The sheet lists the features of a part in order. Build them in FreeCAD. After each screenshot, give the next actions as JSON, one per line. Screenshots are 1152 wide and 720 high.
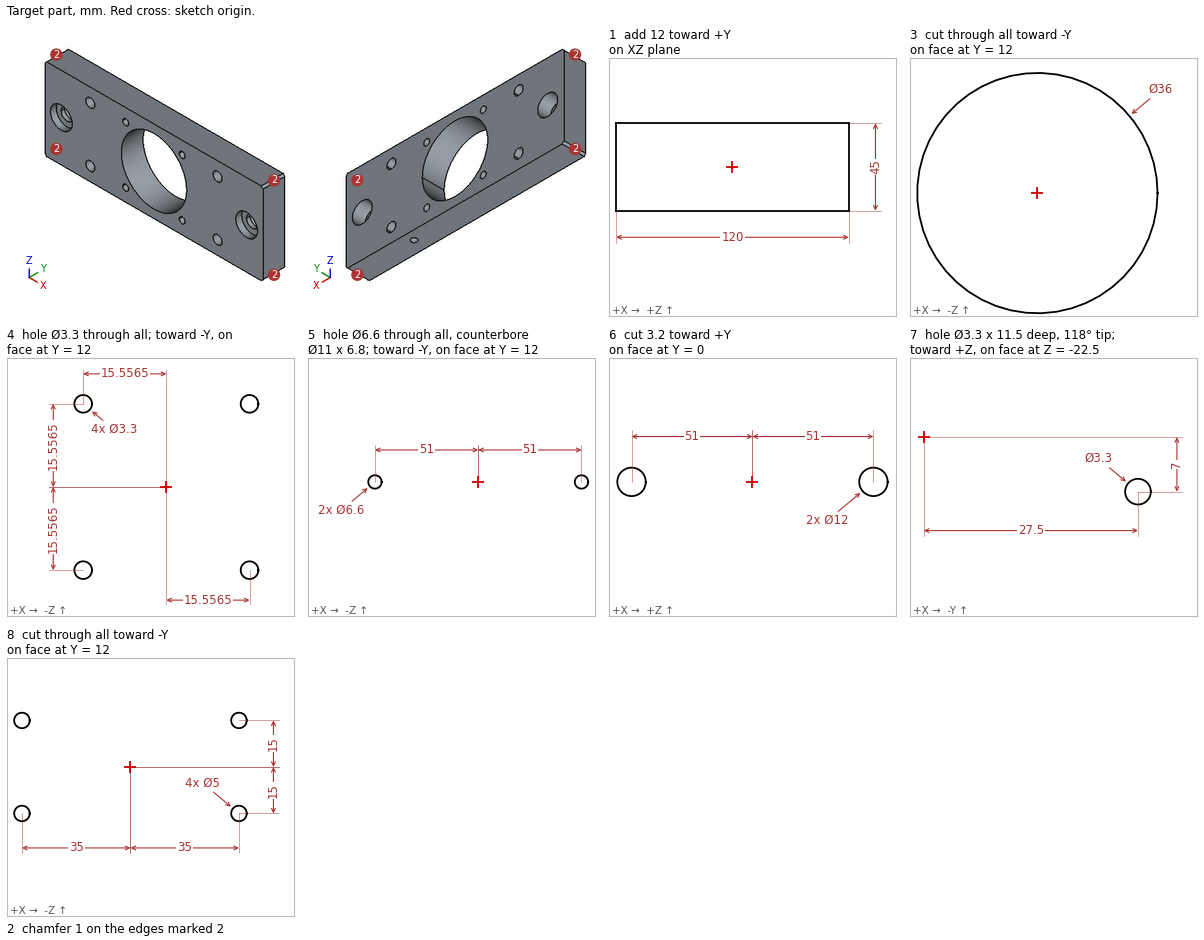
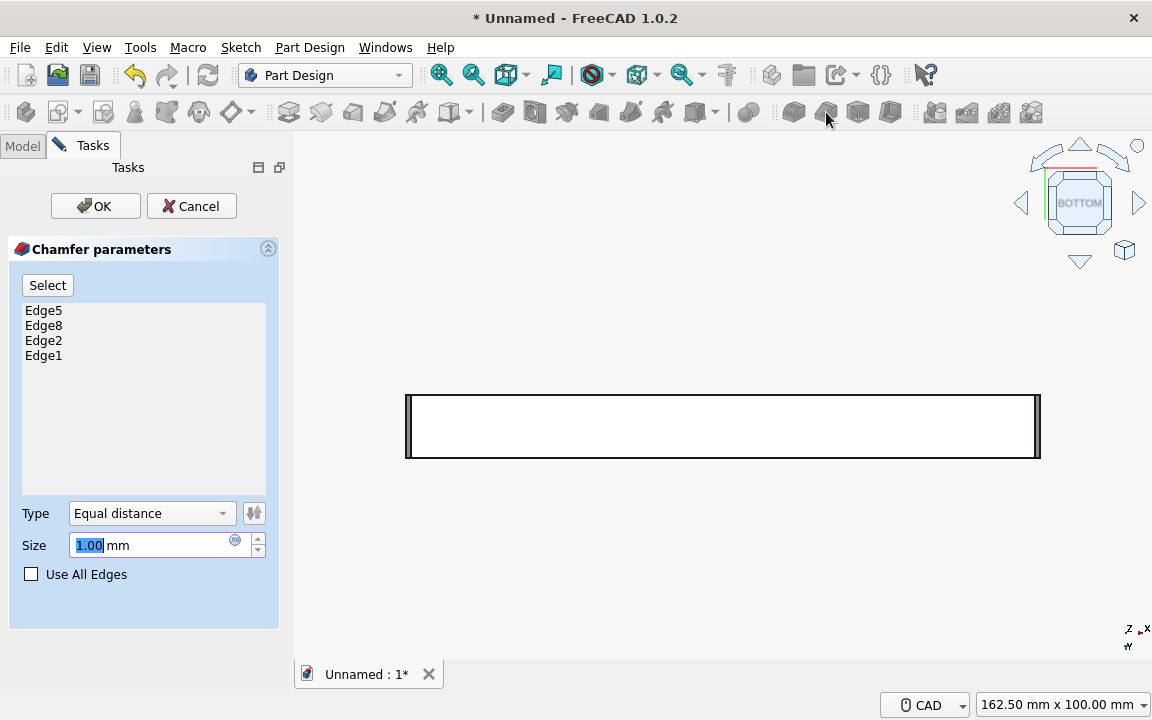
{"action": "type", "text": "1"}
{"action": "key", "text": "Tab"}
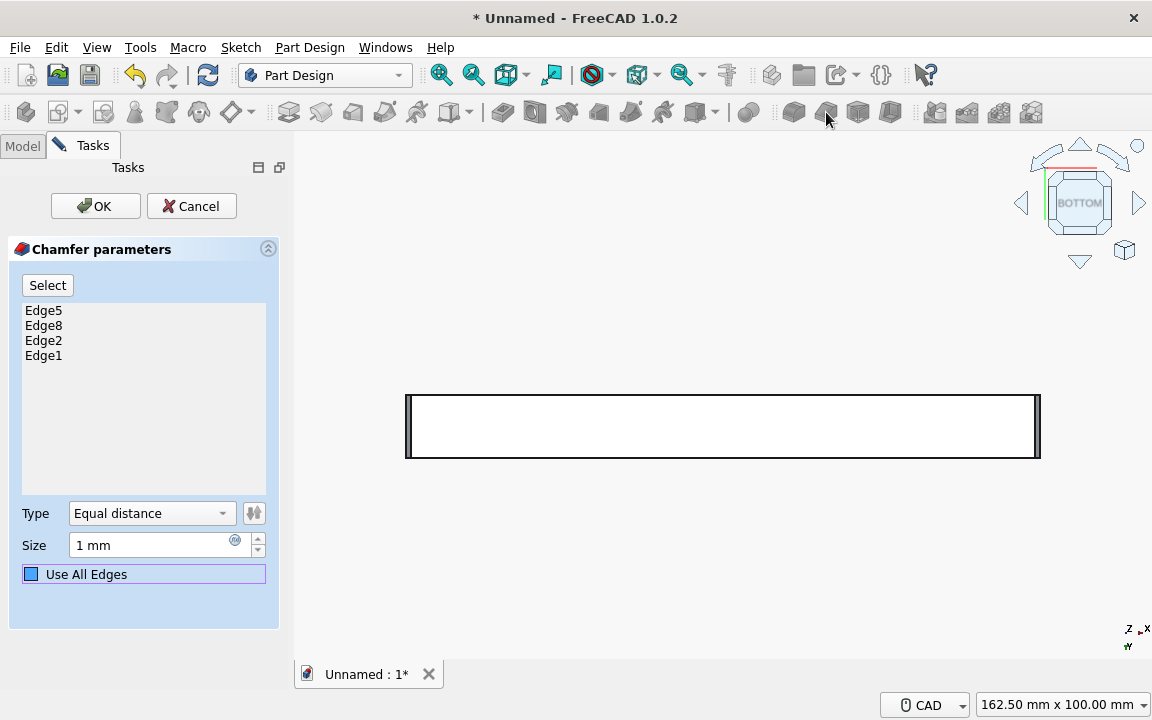
{"action": "left_click", "coordinate": [96, 206]}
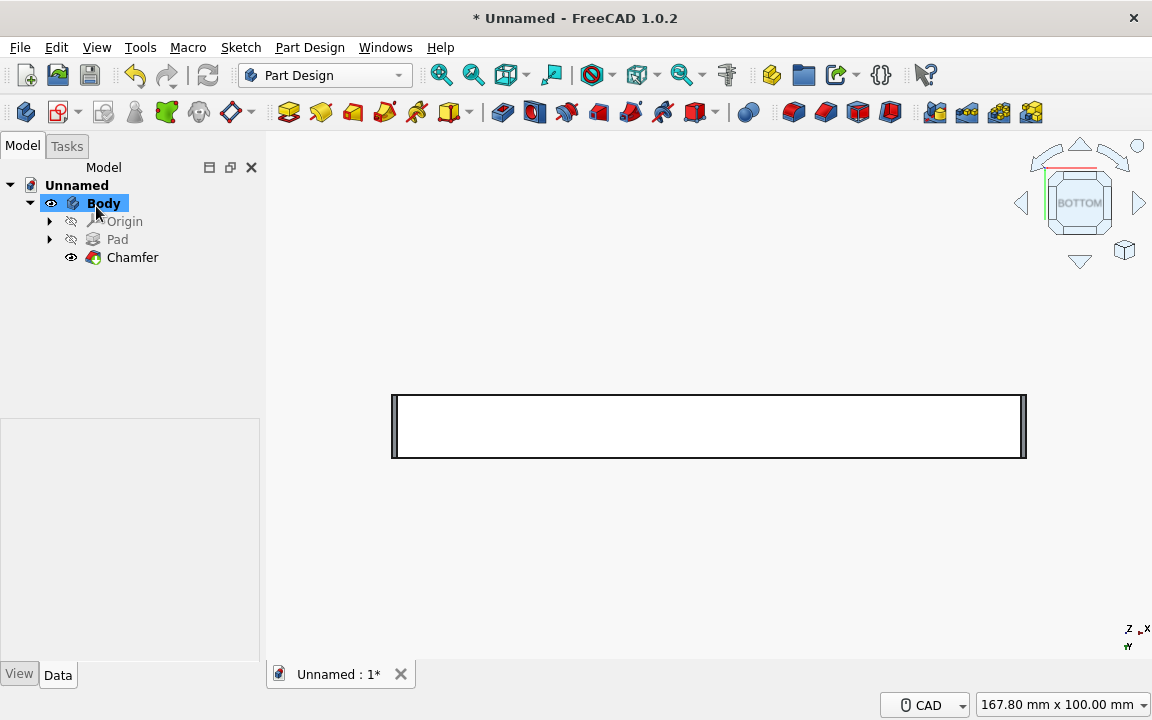
{"action": "key", "text": "4"}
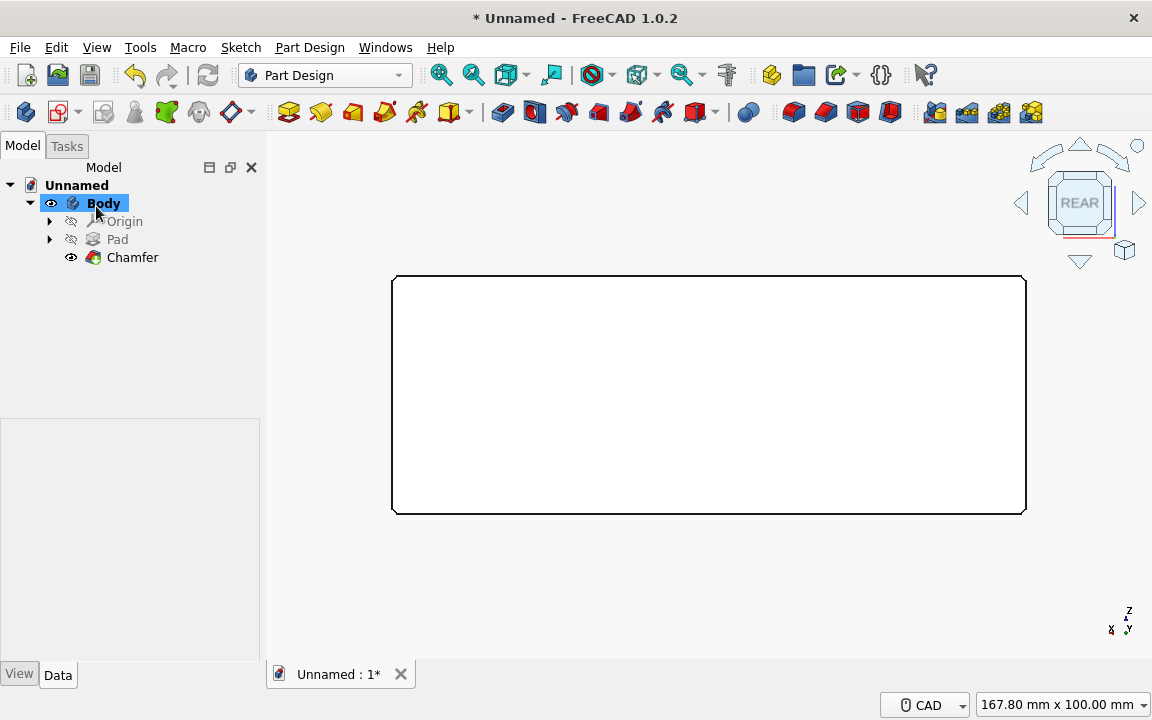
{"action": "left_click", "coordinate": [528, 394]}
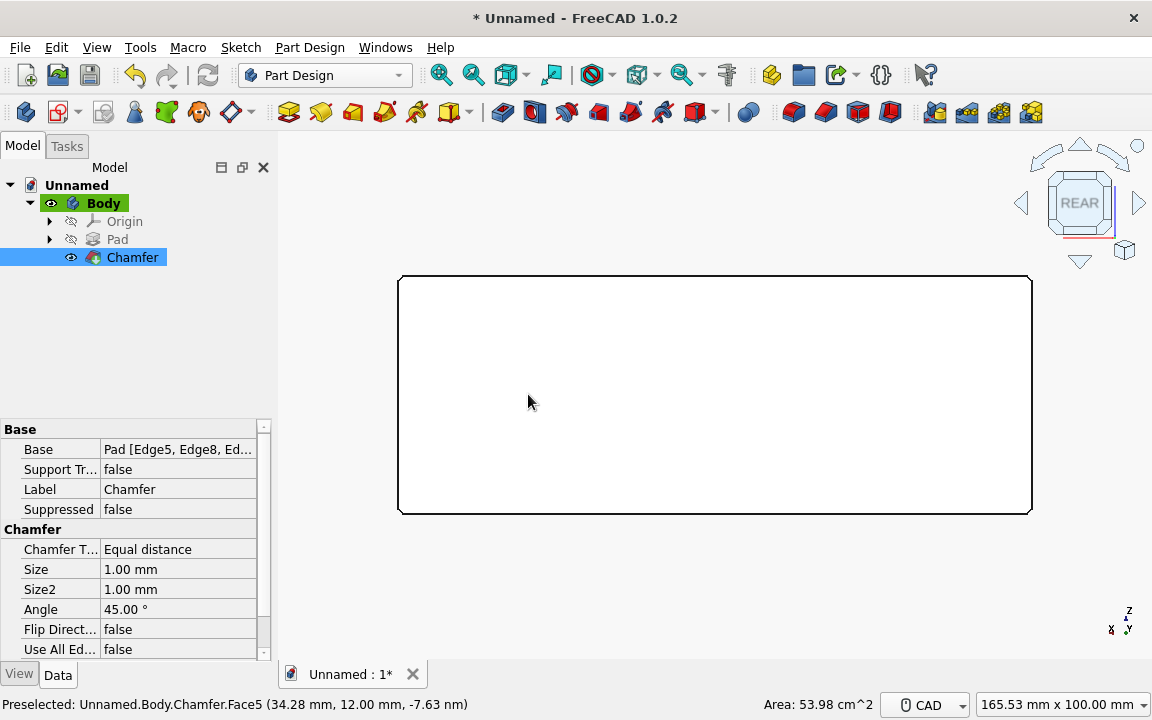
{"action": "left_click", "coordinate": [58, 112]}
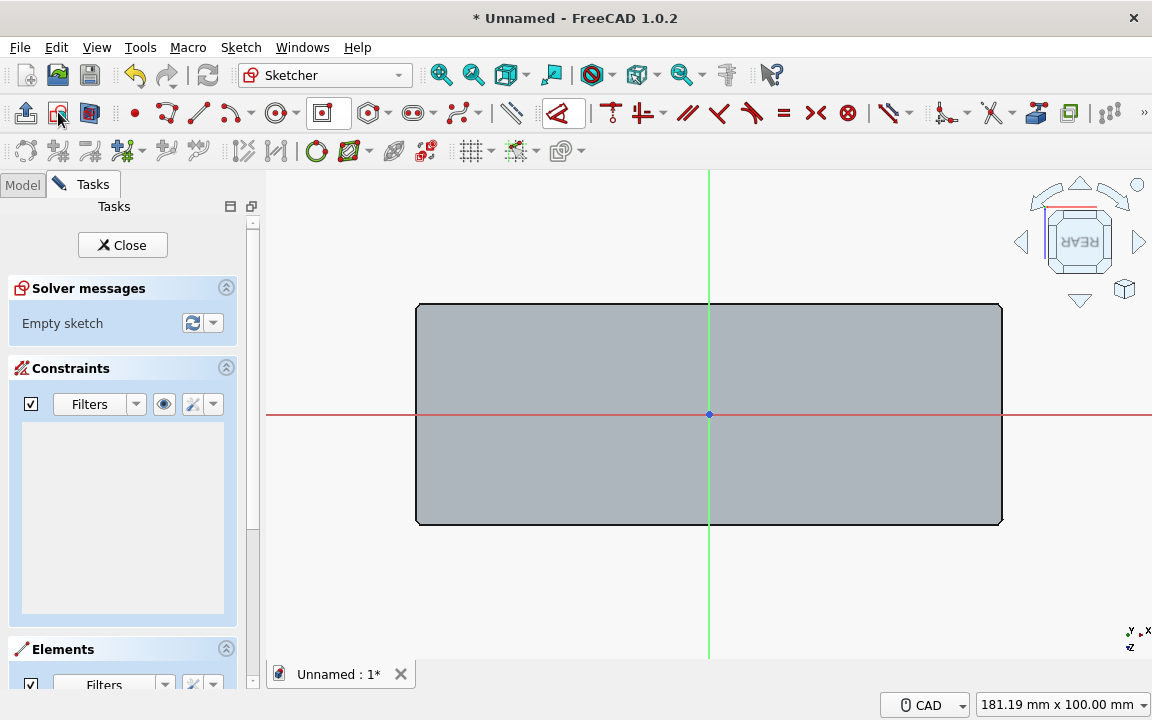
{"action": "scroll", "coordinate": [792, 415], "scroll_direction": "up", "scroll_amount": 3}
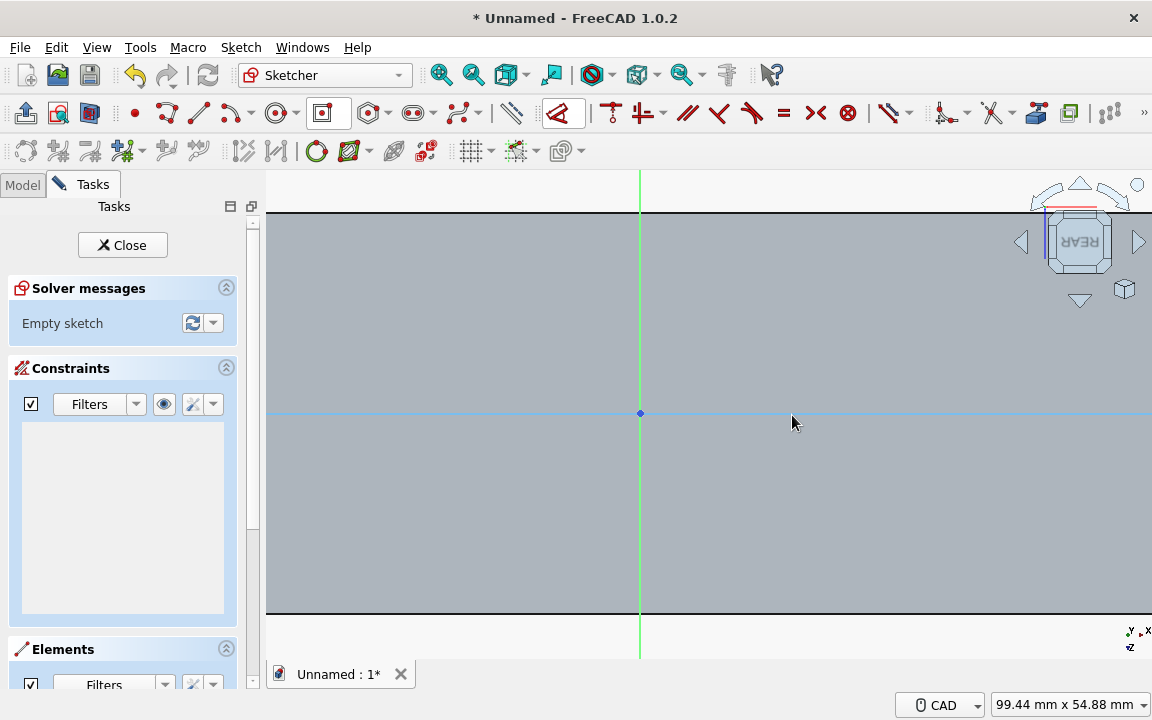
{"action": "left_click", "coordinate": [276, 114]}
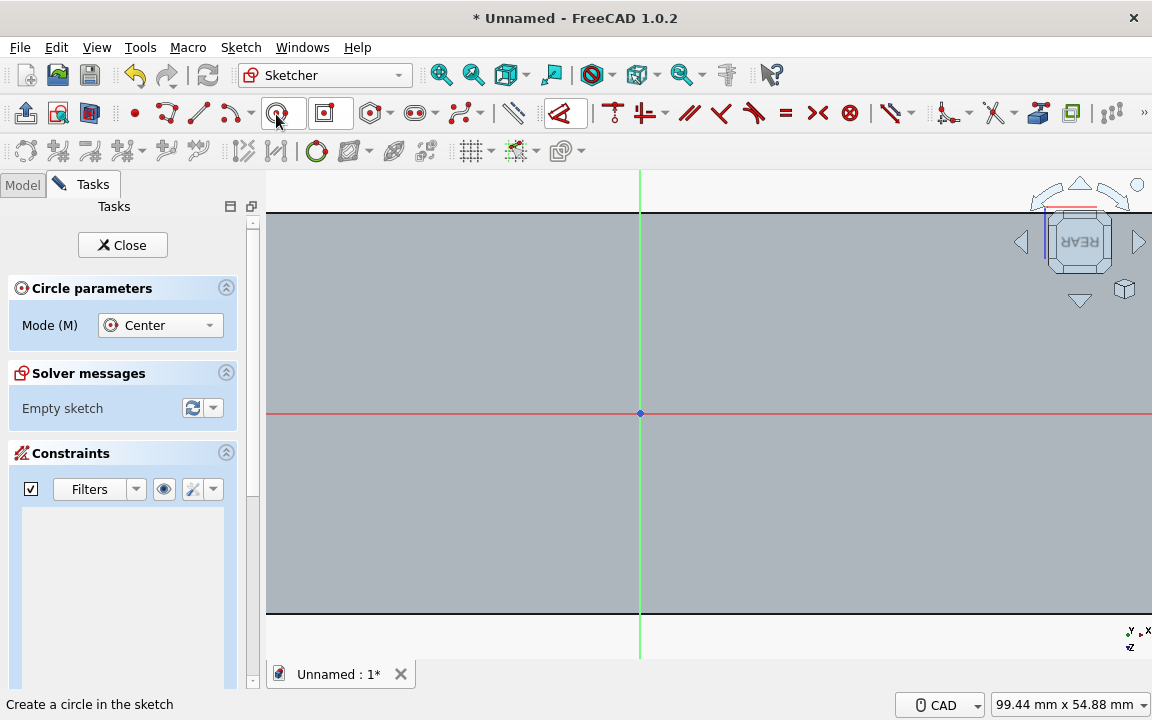
{"action": "left_click", "coordinate": [640, 414]}
{"action": "mouse_move", "coordinate": [754, 300]}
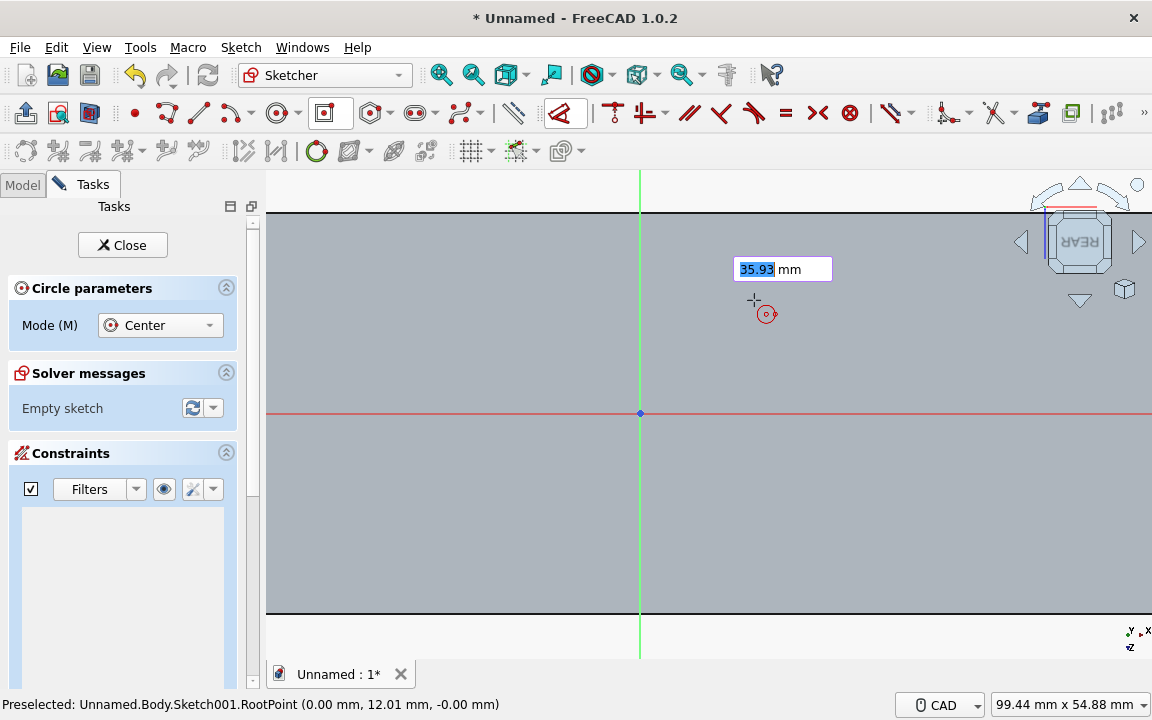
{"action": "type", "text": "36"}
{"action": "key", "text": "Return"}
{"action": "key", "text": "Escape"}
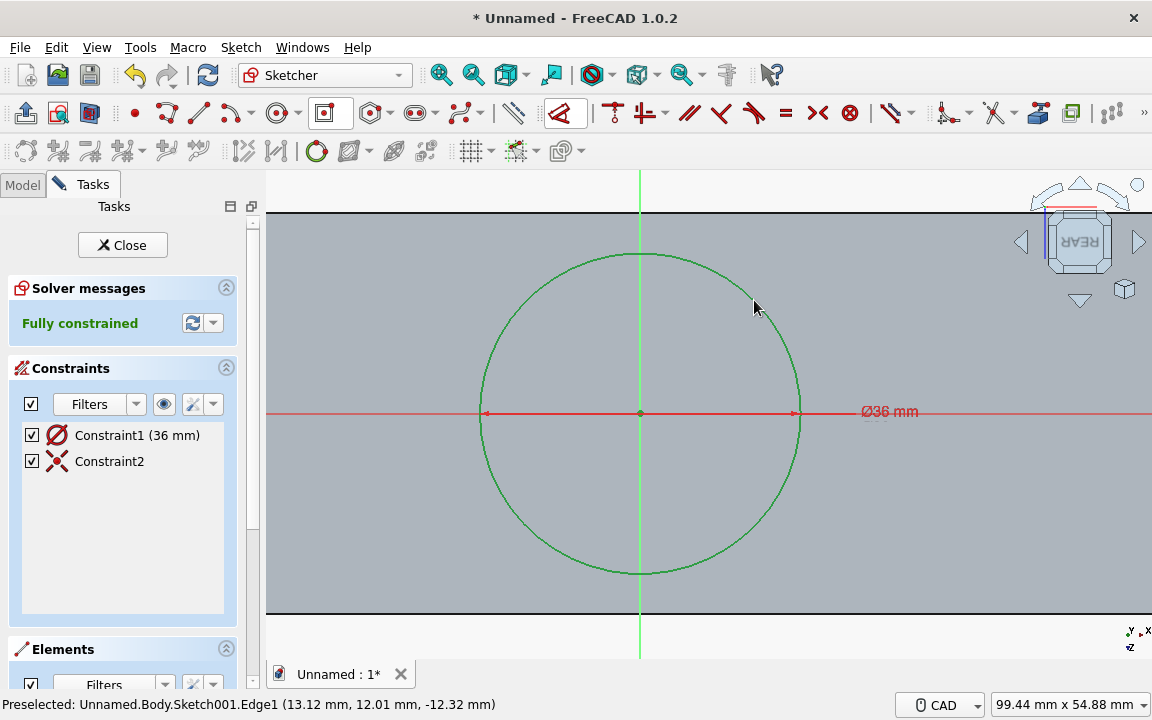
{"action": "left_click", "coordinate": [123, 245]}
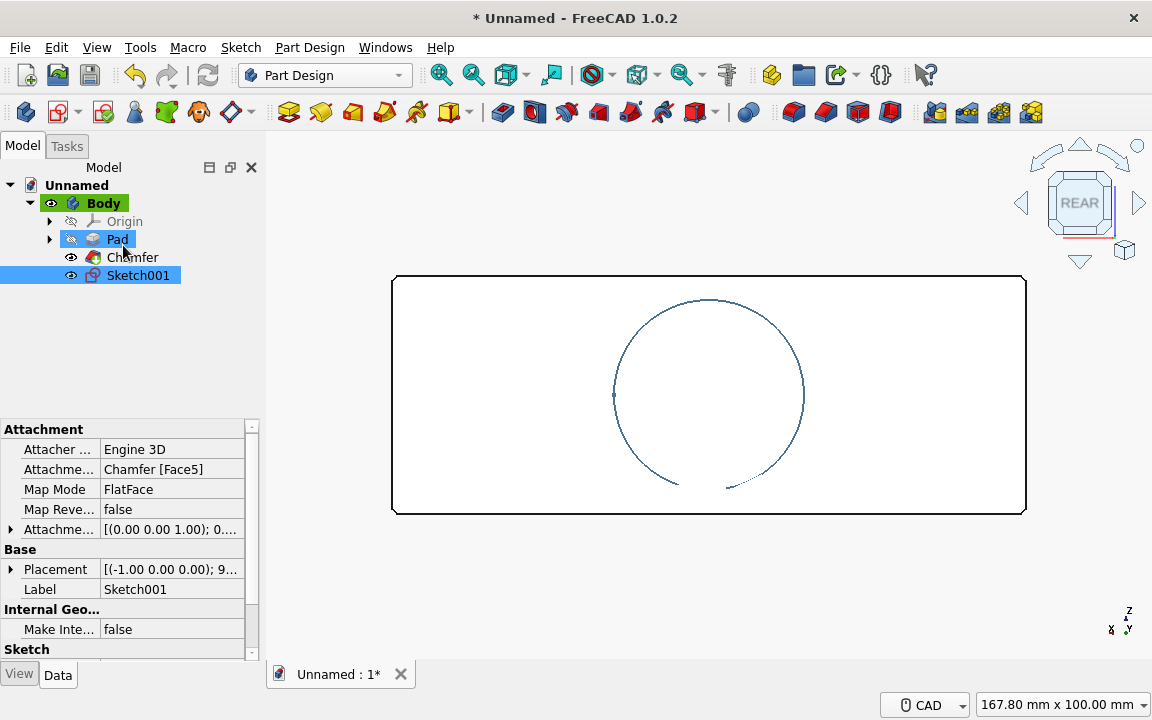
{"action": "left_click", "coordinate": [504, 112]}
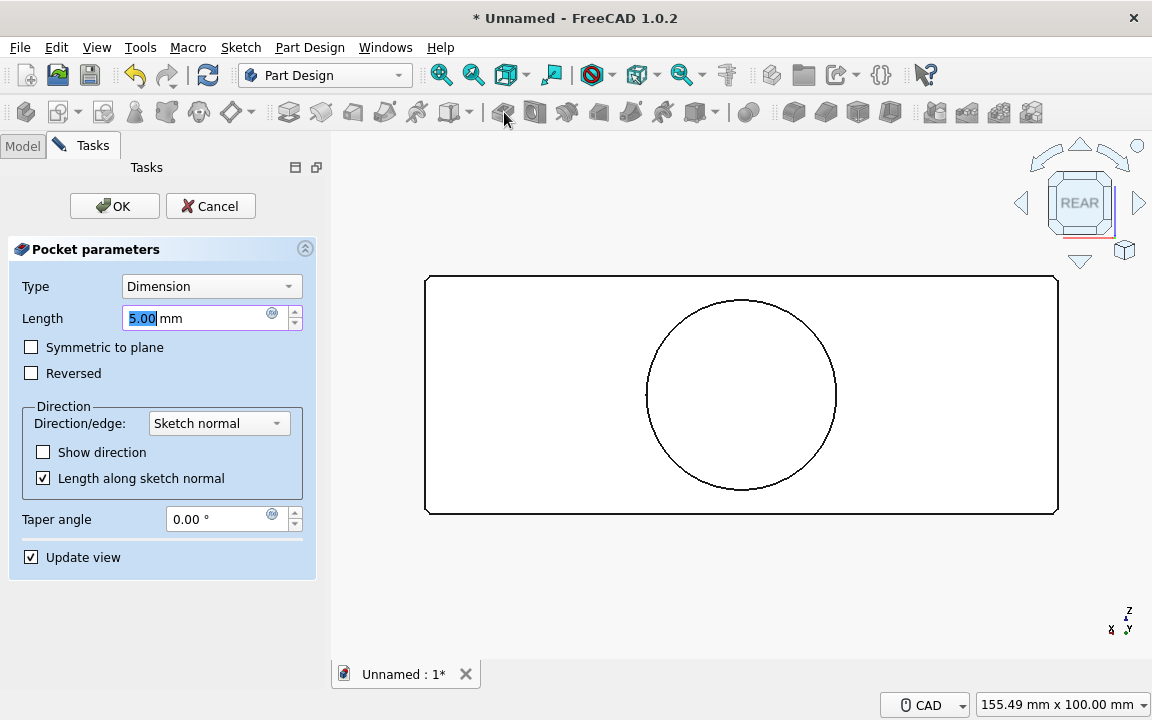
{"action": "left_click", "coordinate": [212, 286]}